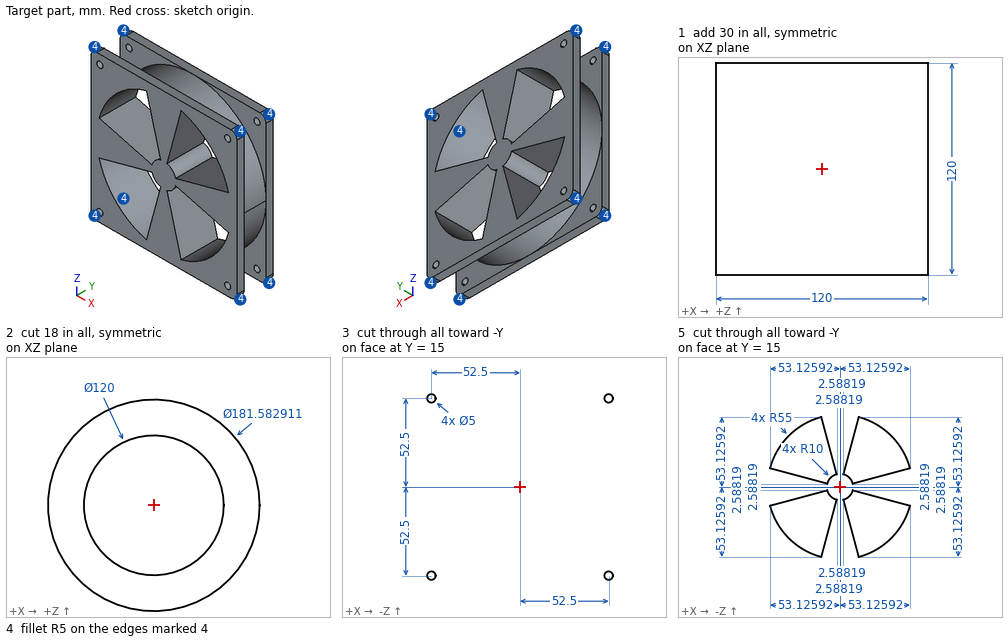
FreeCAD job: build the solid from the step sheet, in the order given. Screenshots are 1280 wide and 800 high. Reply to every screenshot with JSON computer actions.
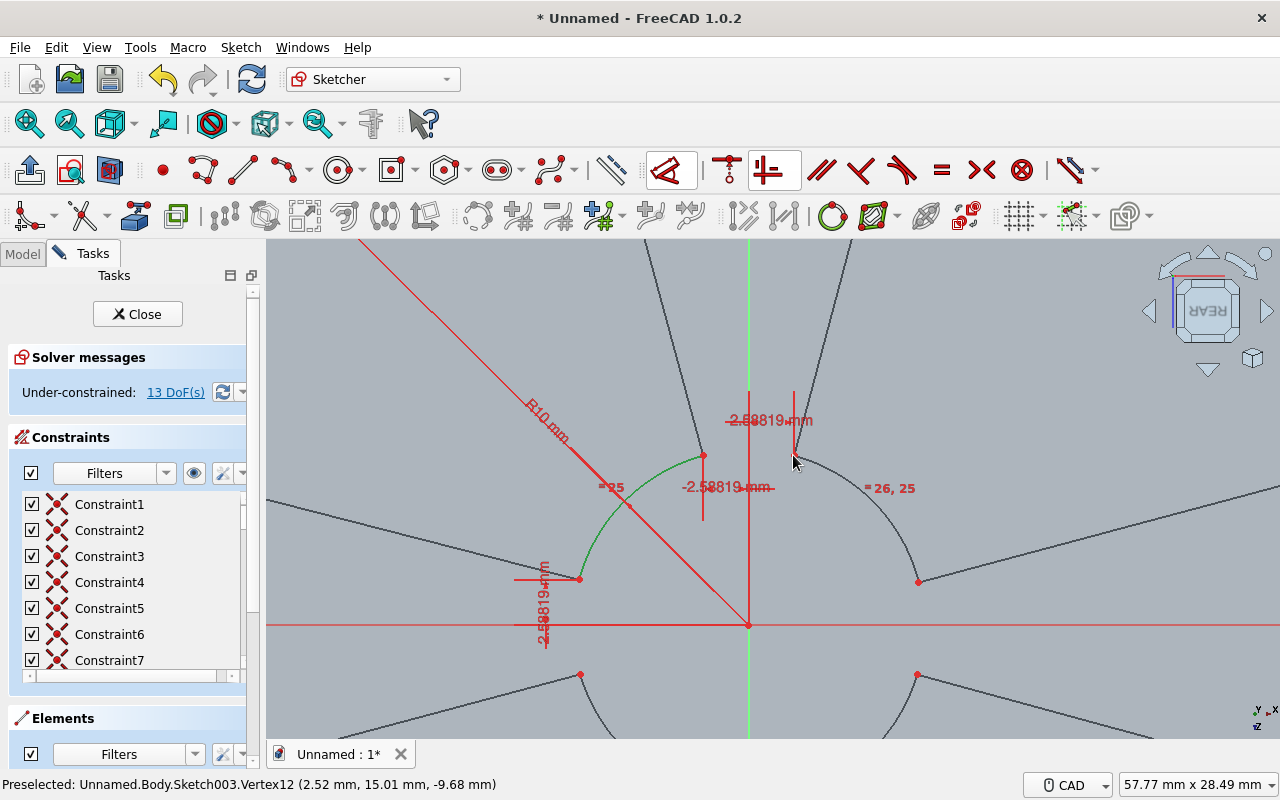
{"action": "left_click", "coordinate": [919, 582]}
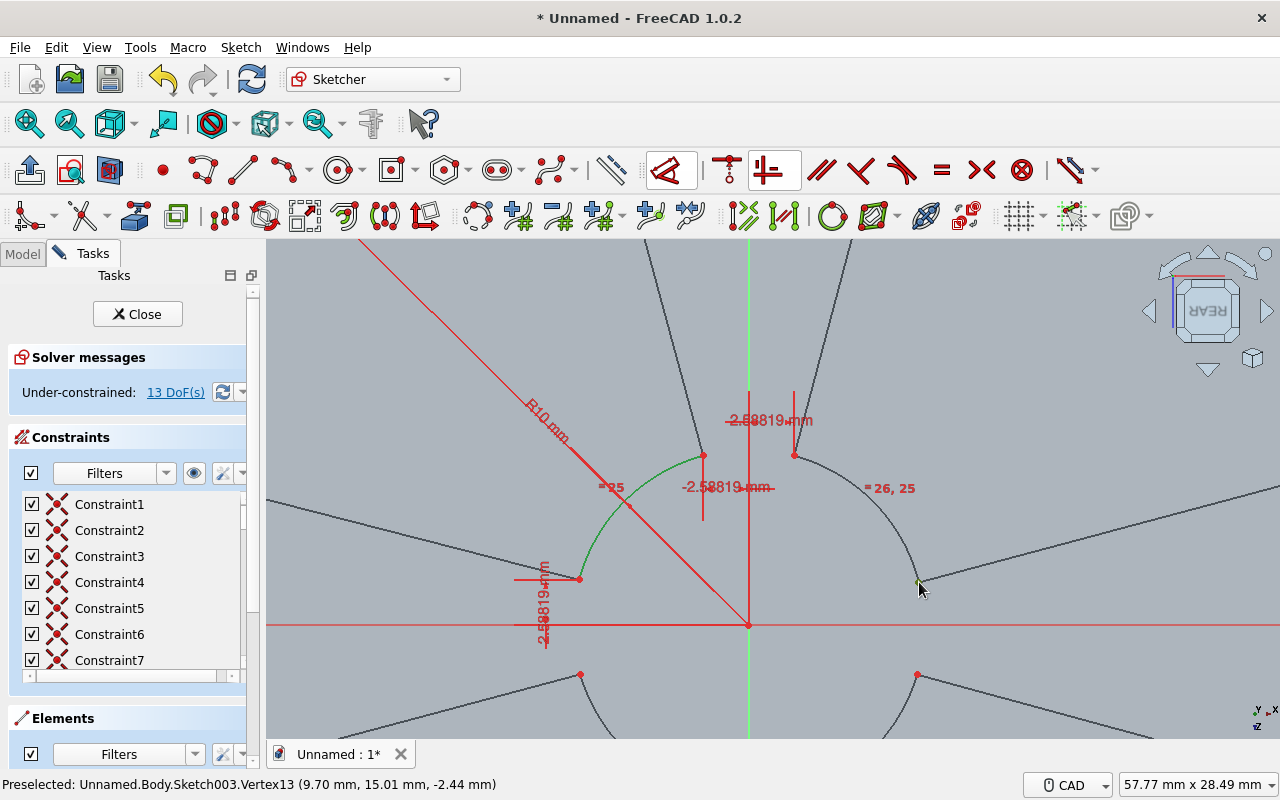
{"action": "key", "text": "i"}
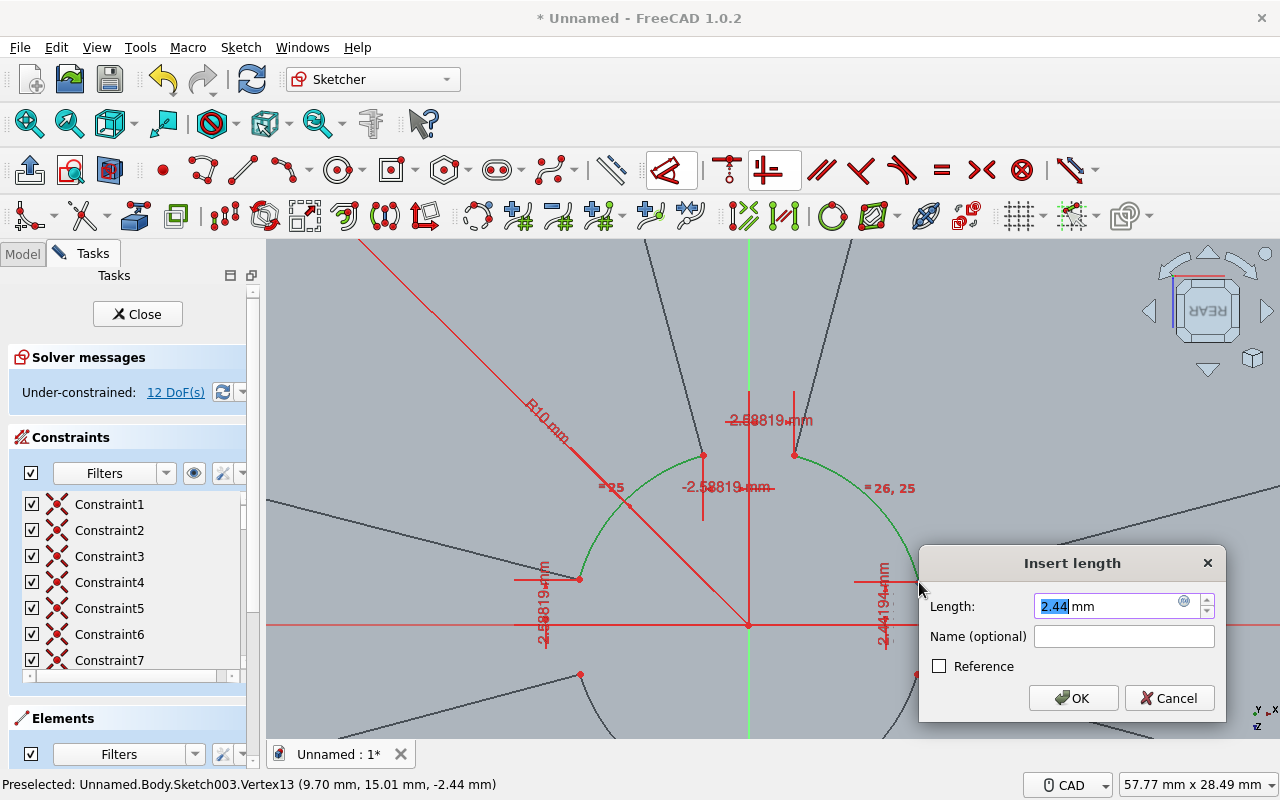
{"action": "type", "text": "2.58819"}
{"action": "key", "text": "Return"}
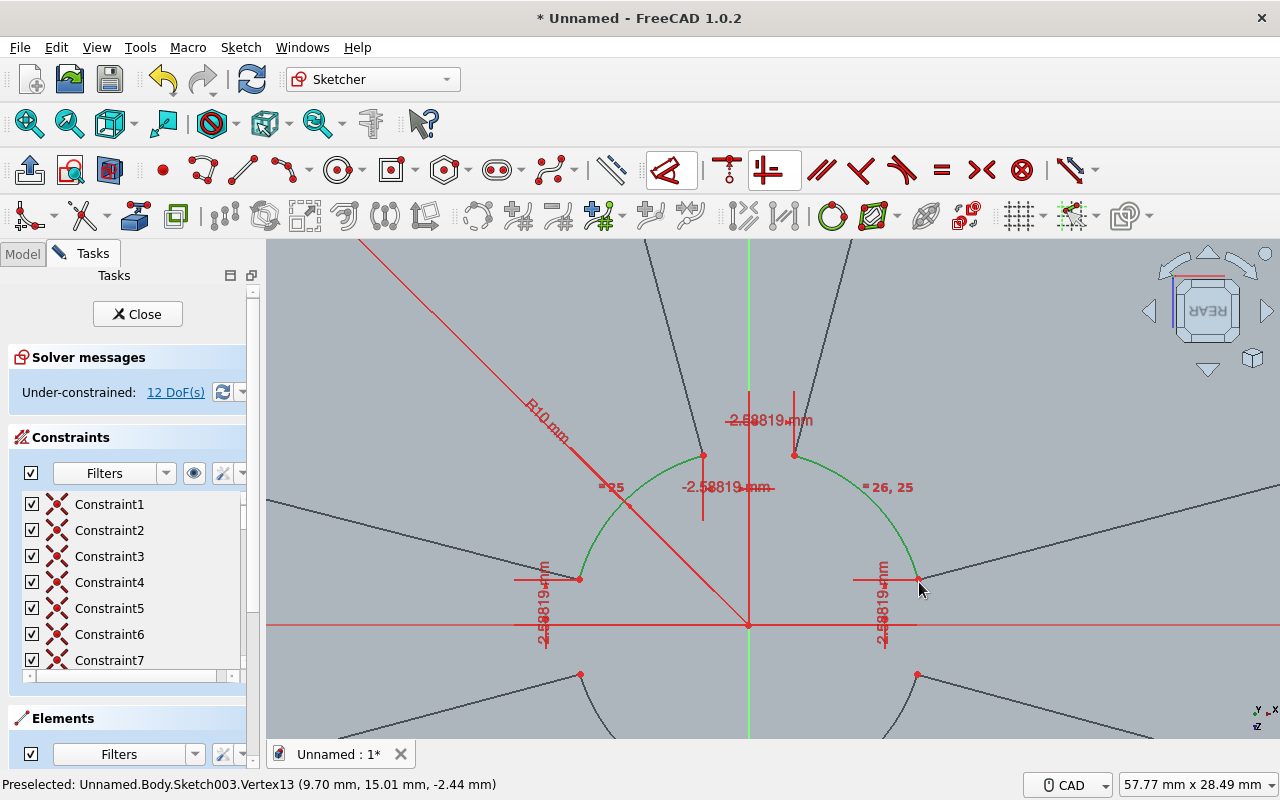
{"action": "scroll", "coordinate": [696, 462], "scroll_direction": "down", "scroll_amount": 9}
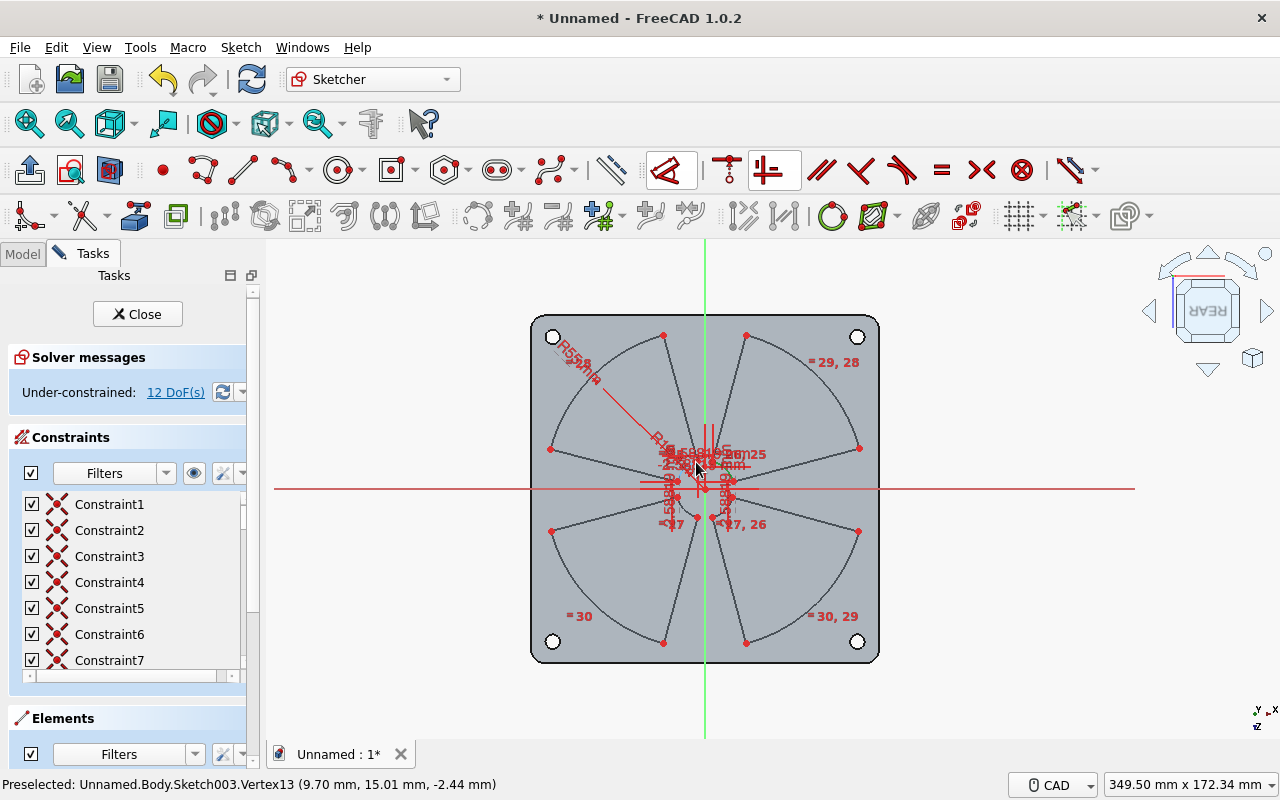
{"action": "scroll", "coordinate": [712, 517], "scroll_direction": "up", "scroll_amount": 9}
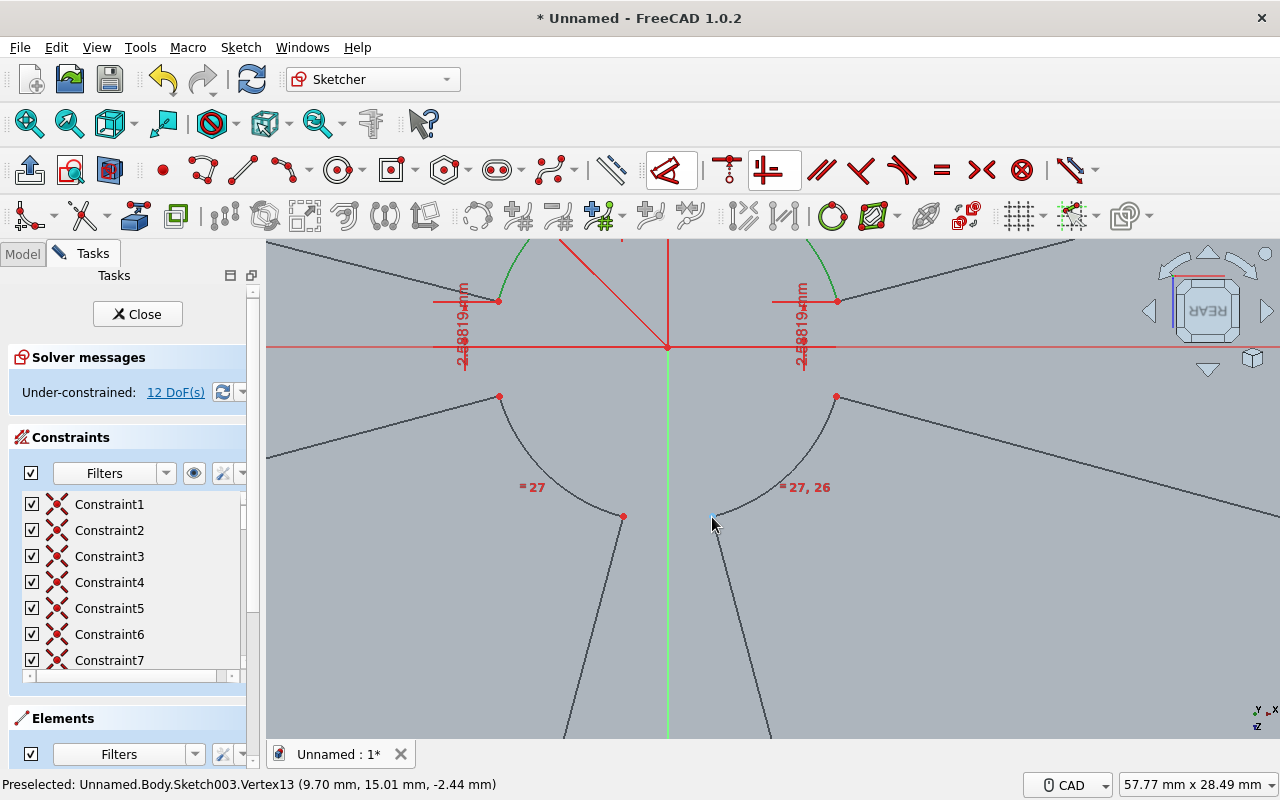
{"action": "left_click", "coordinate": [712, 517]}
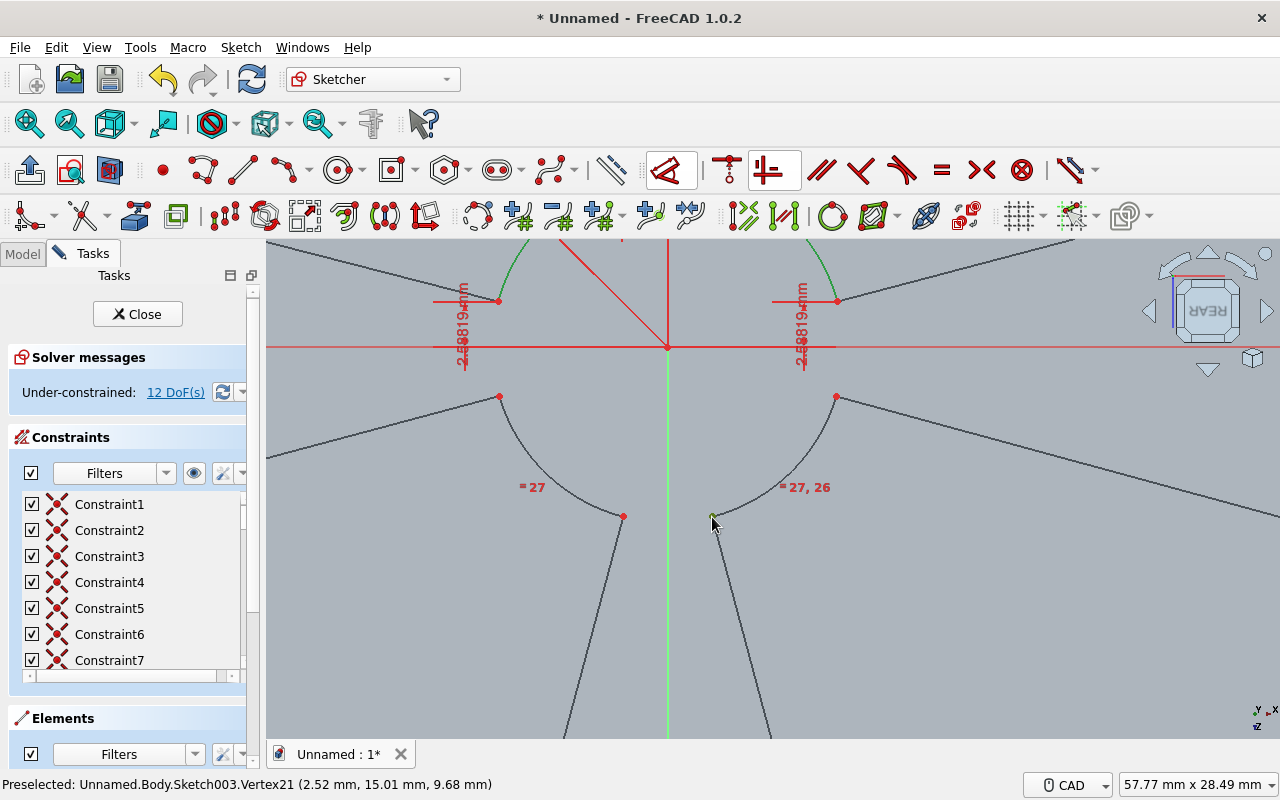
{"action": "key", "text": "l"}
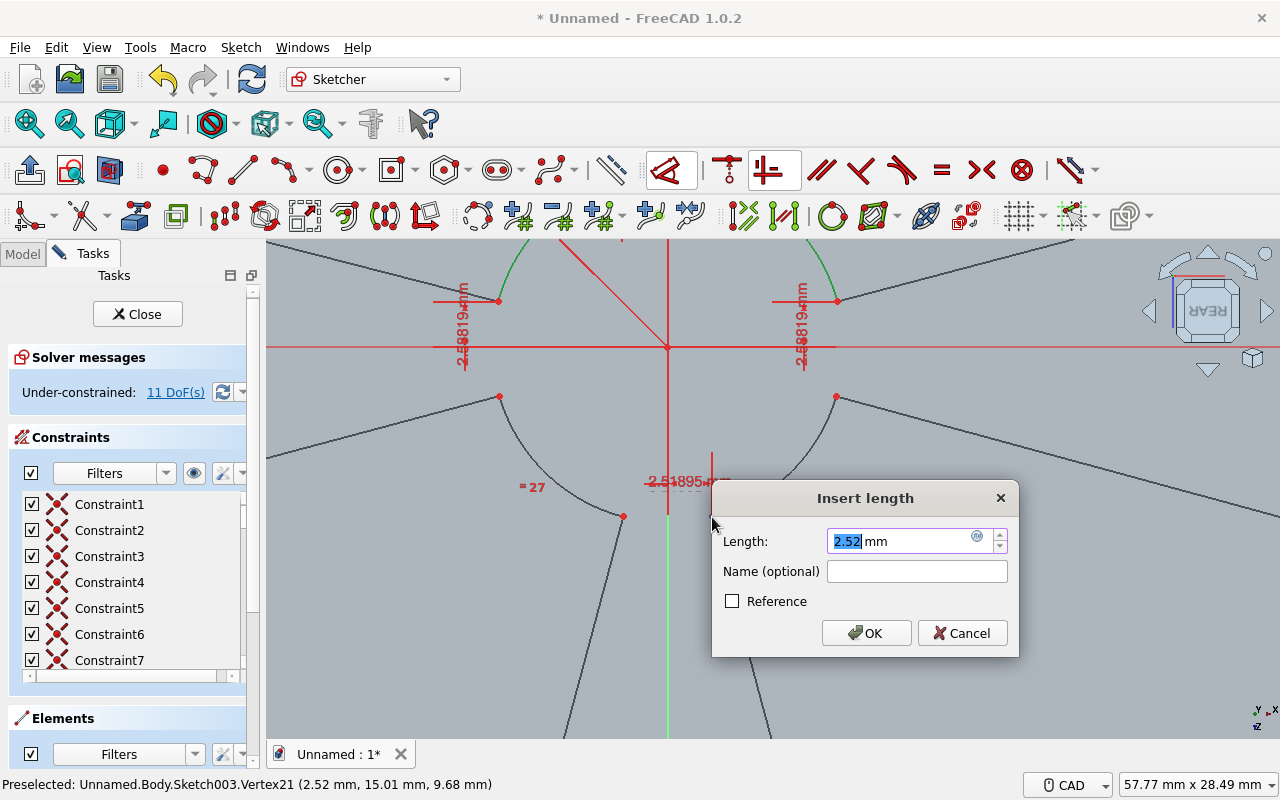
{"action": "type", "text": "2.58819"}
{"action": "key", "text": "Return"}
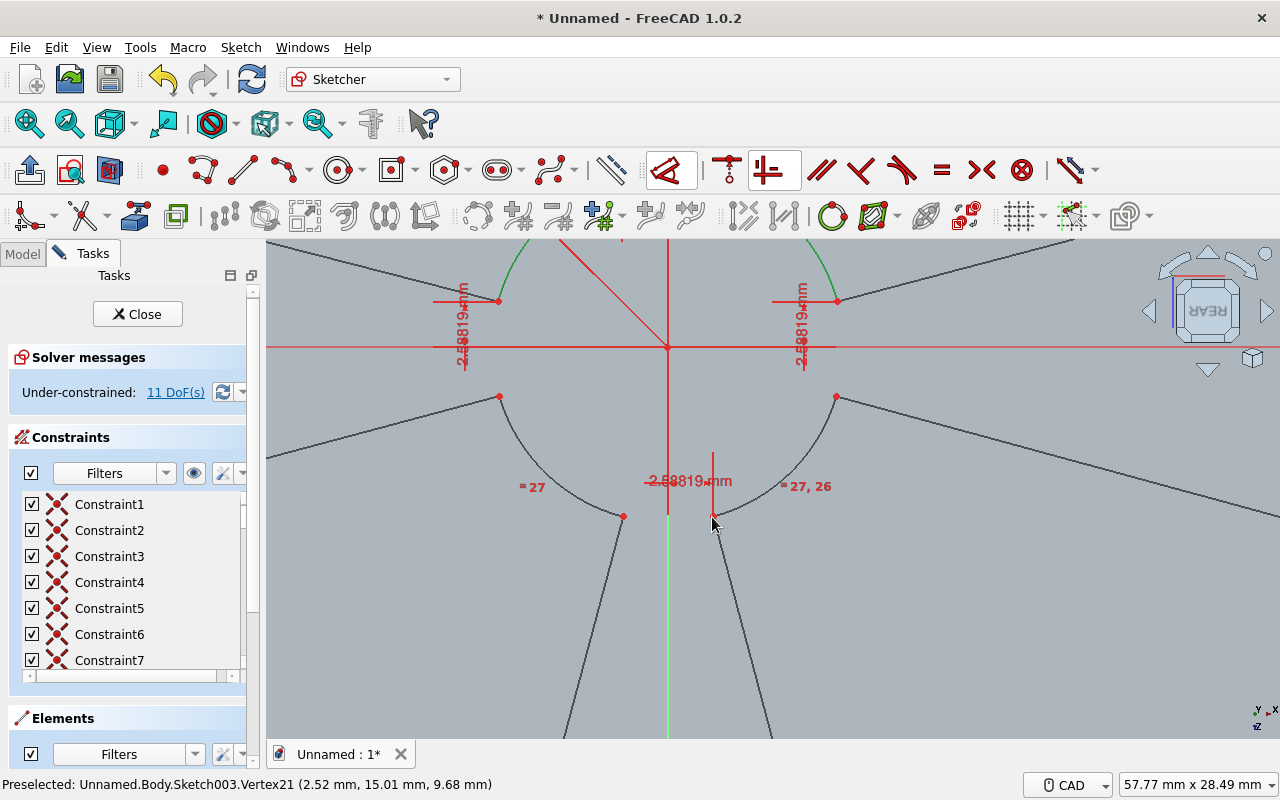
{"action": "left_click", "coordinate": [836, 396]}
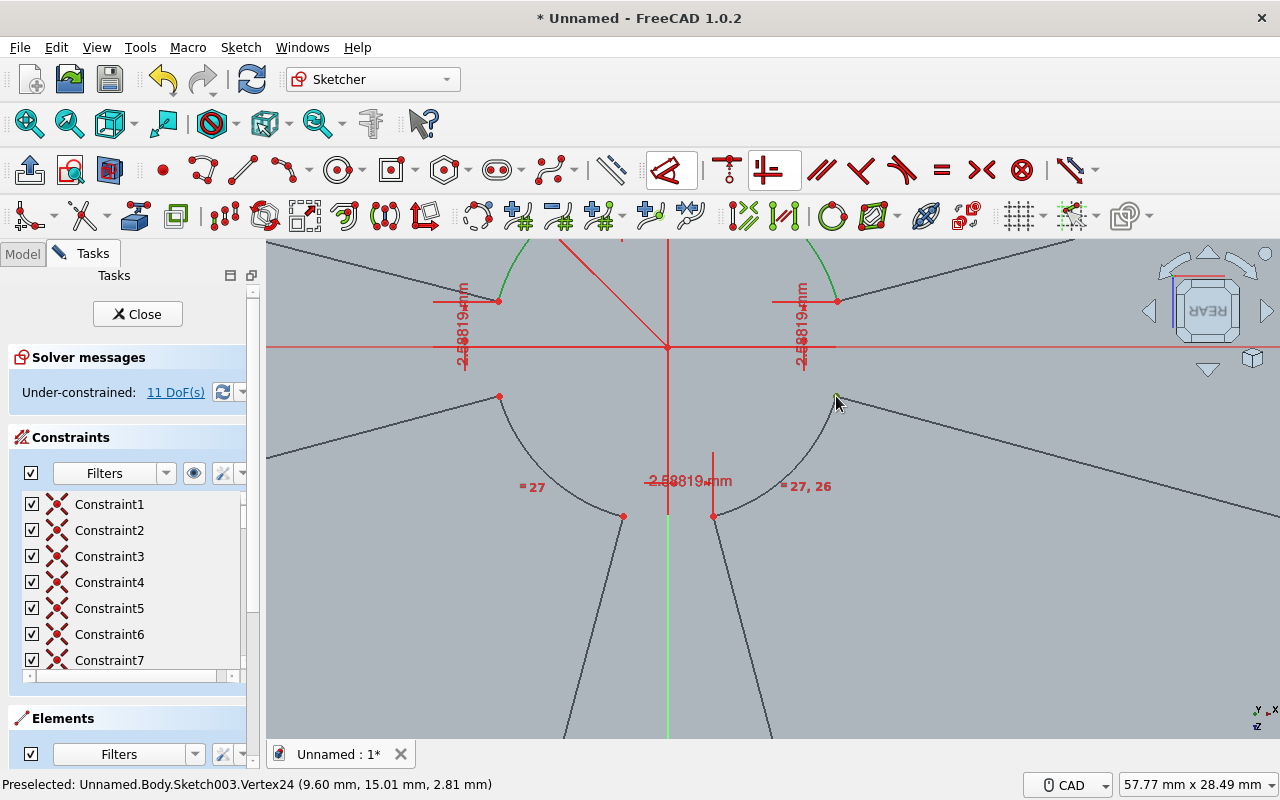
{"action": "key", "text": "i"}